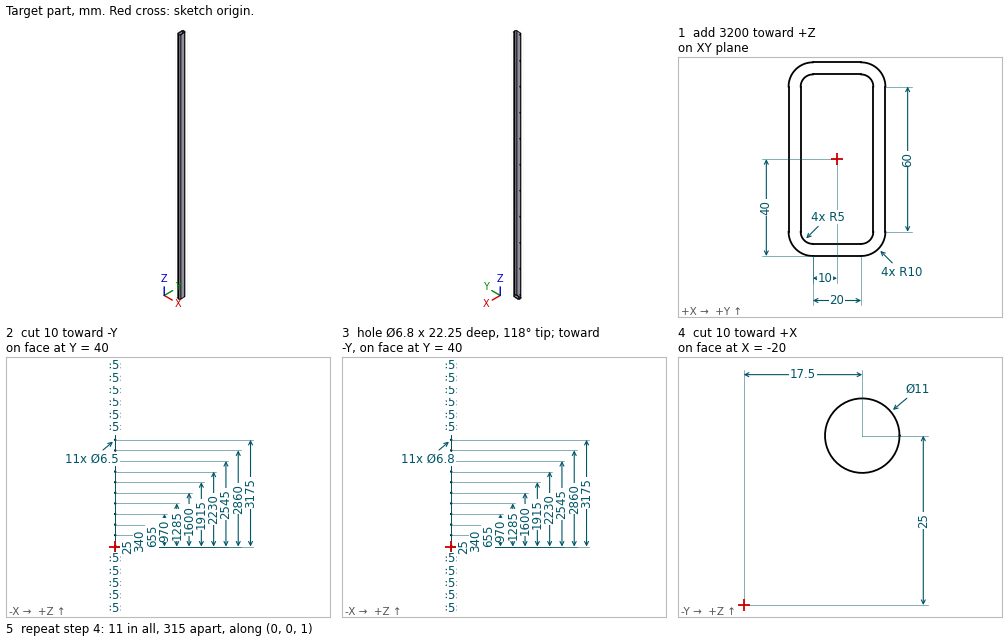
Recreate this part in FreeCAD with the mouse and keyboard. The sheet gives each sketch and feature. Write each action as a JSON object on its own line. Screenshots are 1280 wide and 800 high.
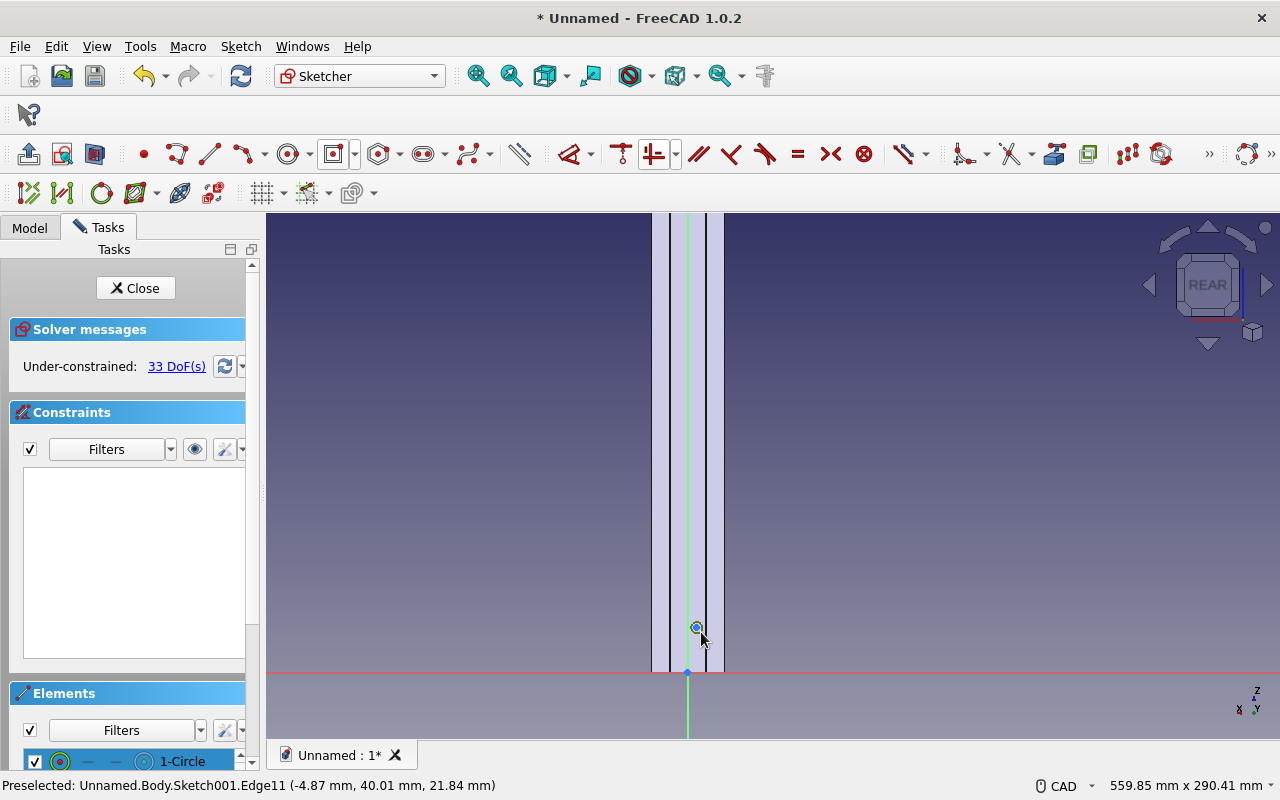
{"action": "key", "text": "e"}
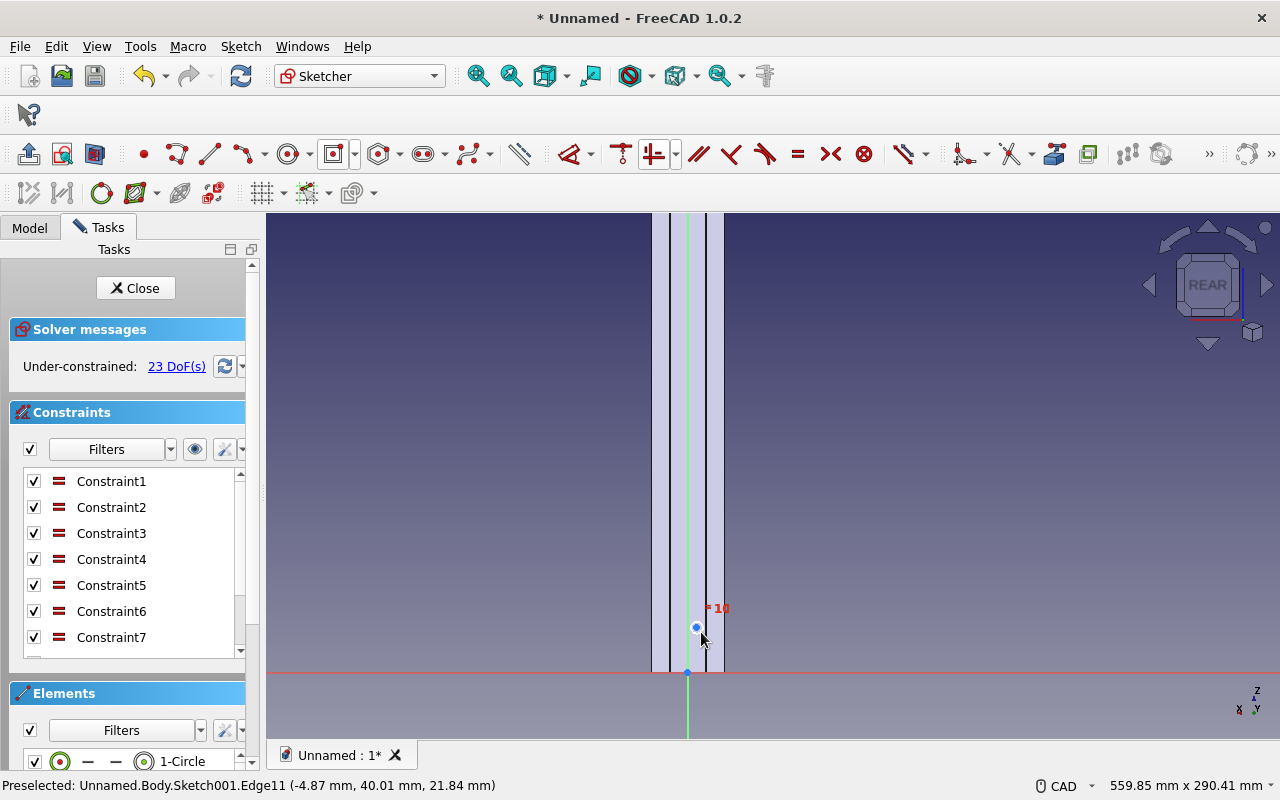
{"action": "left_click", "coordinate": [568, 154]}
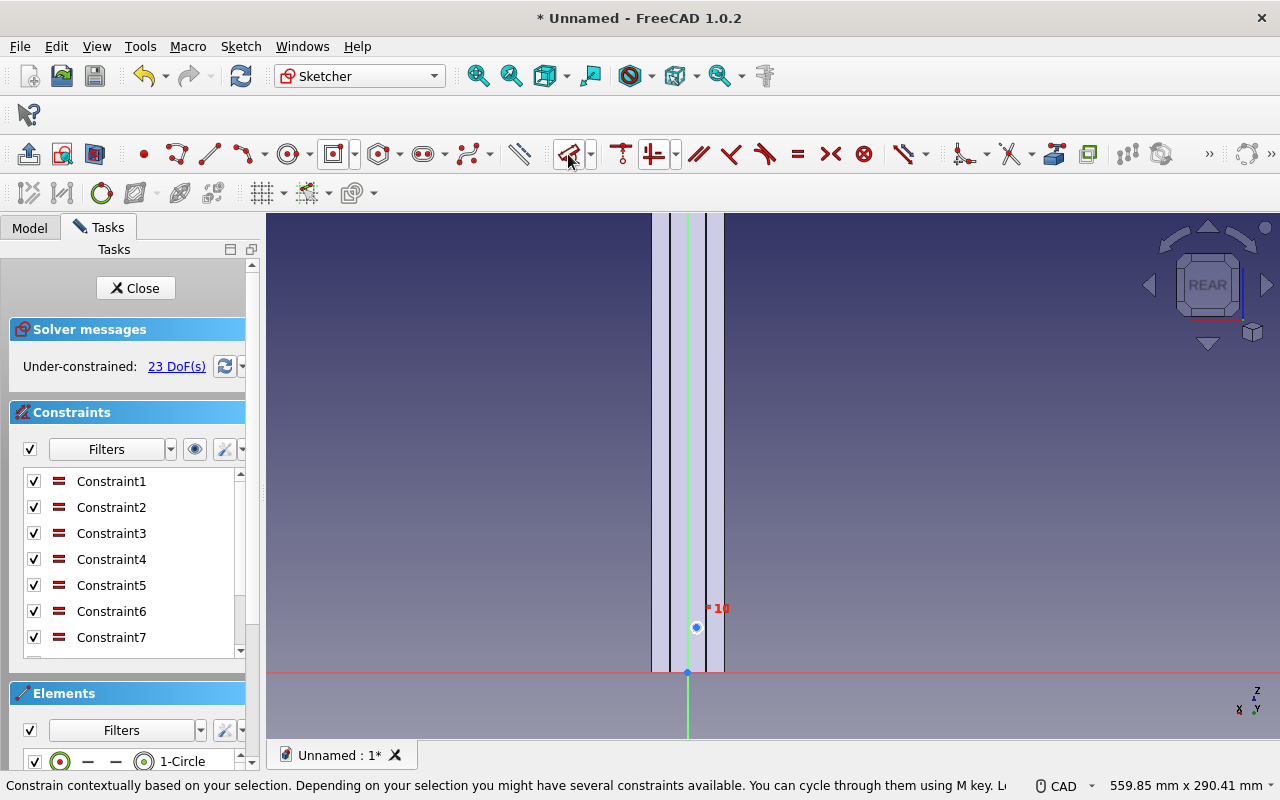
{"action": "scroll", "coordinate": [705, 650], "scroll_direction": "down", "scroll_amount": 14}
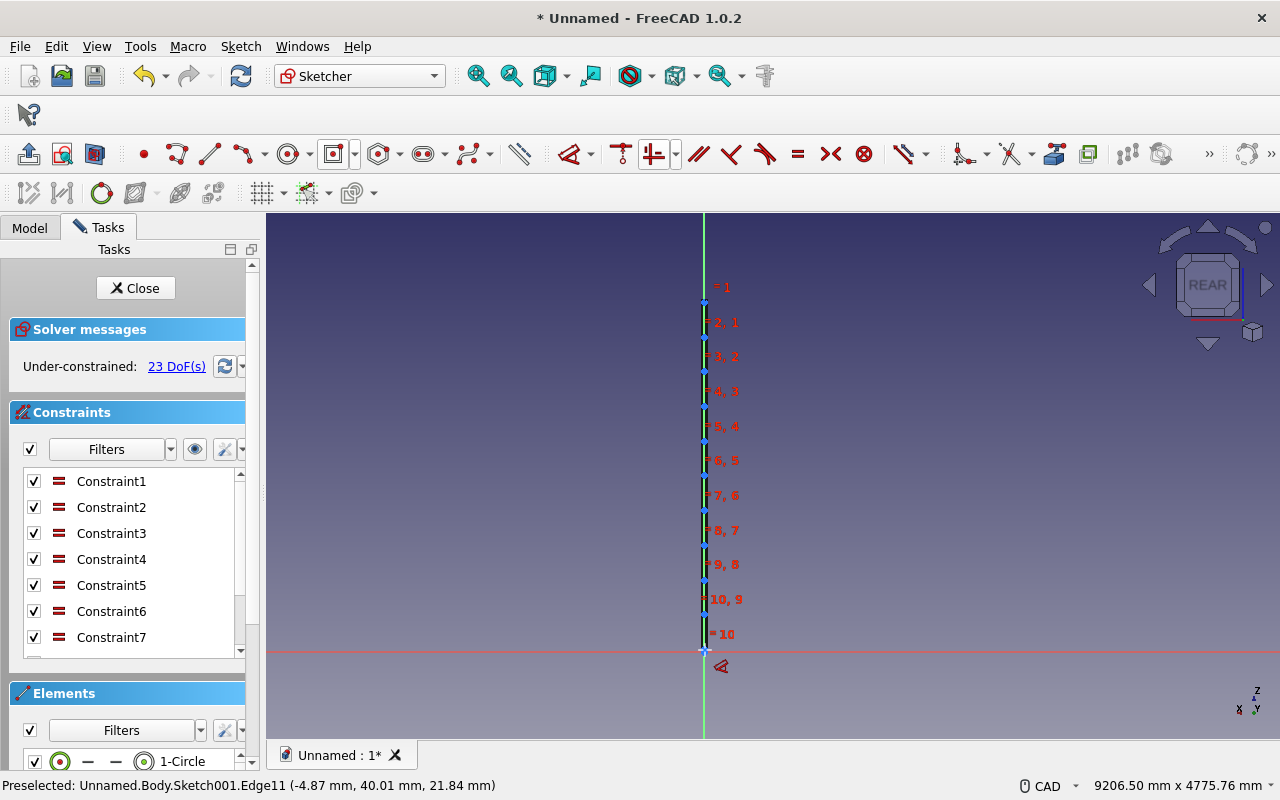
{"action": "scroll", "coordinate": [705, 303], "scroll_direction": "up", "scroll_amount": 21}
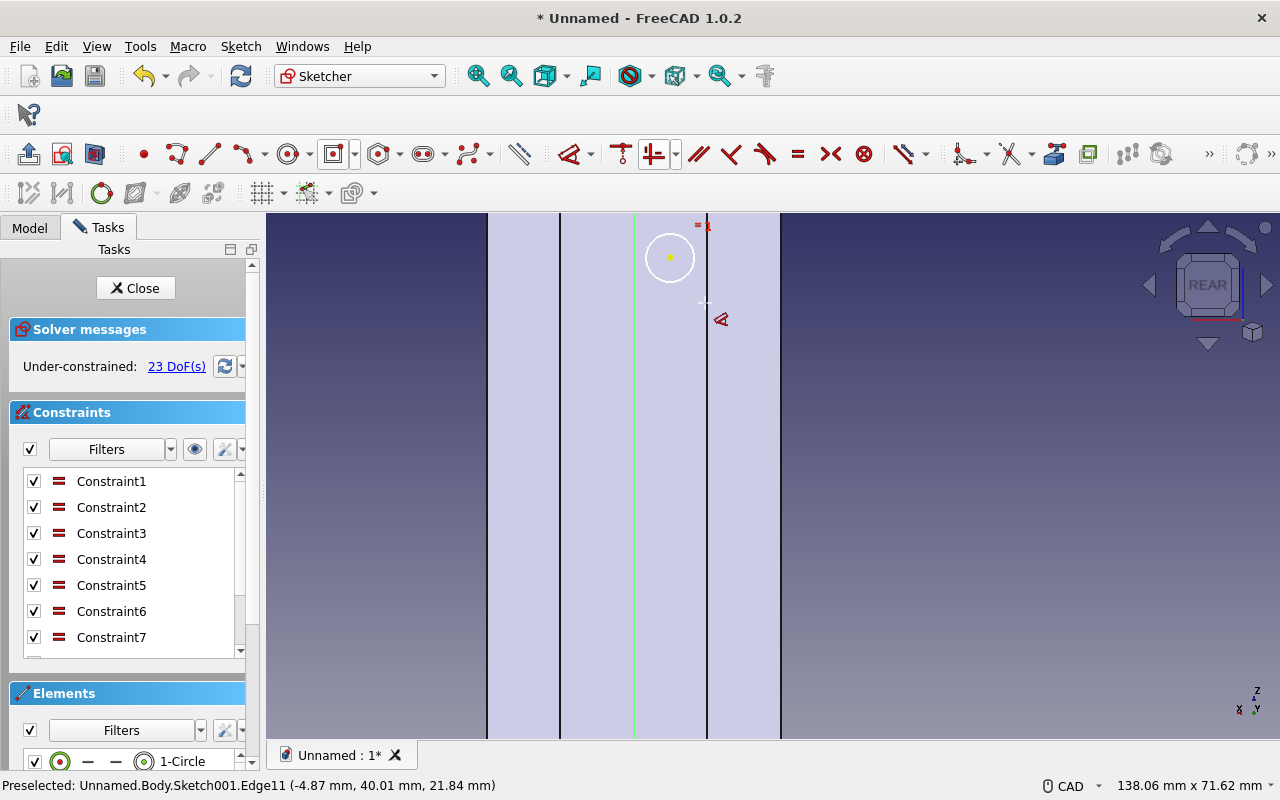
{"action": "left_click", "coordinate": [687, 275]}
{"action": "left_click", "coordinate": [710, 298]}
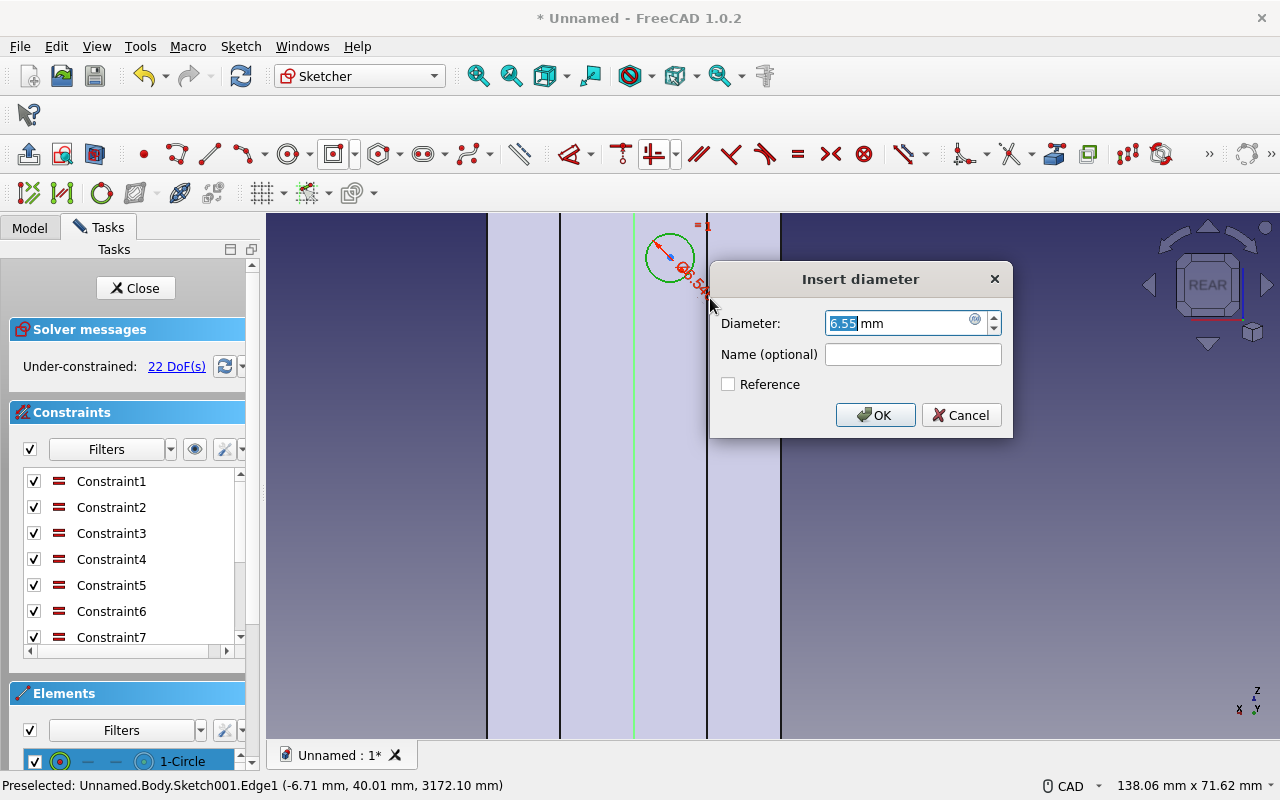
{"action": "type", "text": "6.5"}
{"action": "key", "text": "Return"}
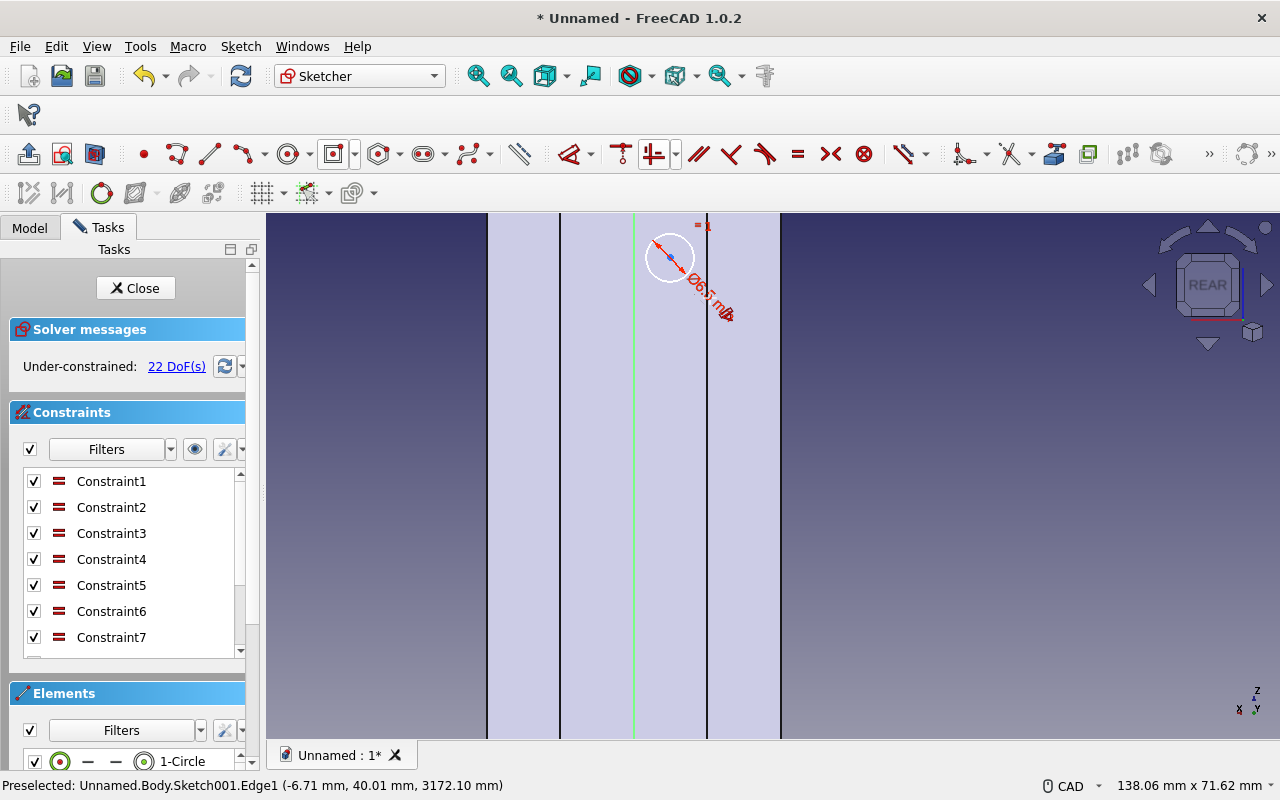
{"action": "left_click", "coordinate": [670, 258]}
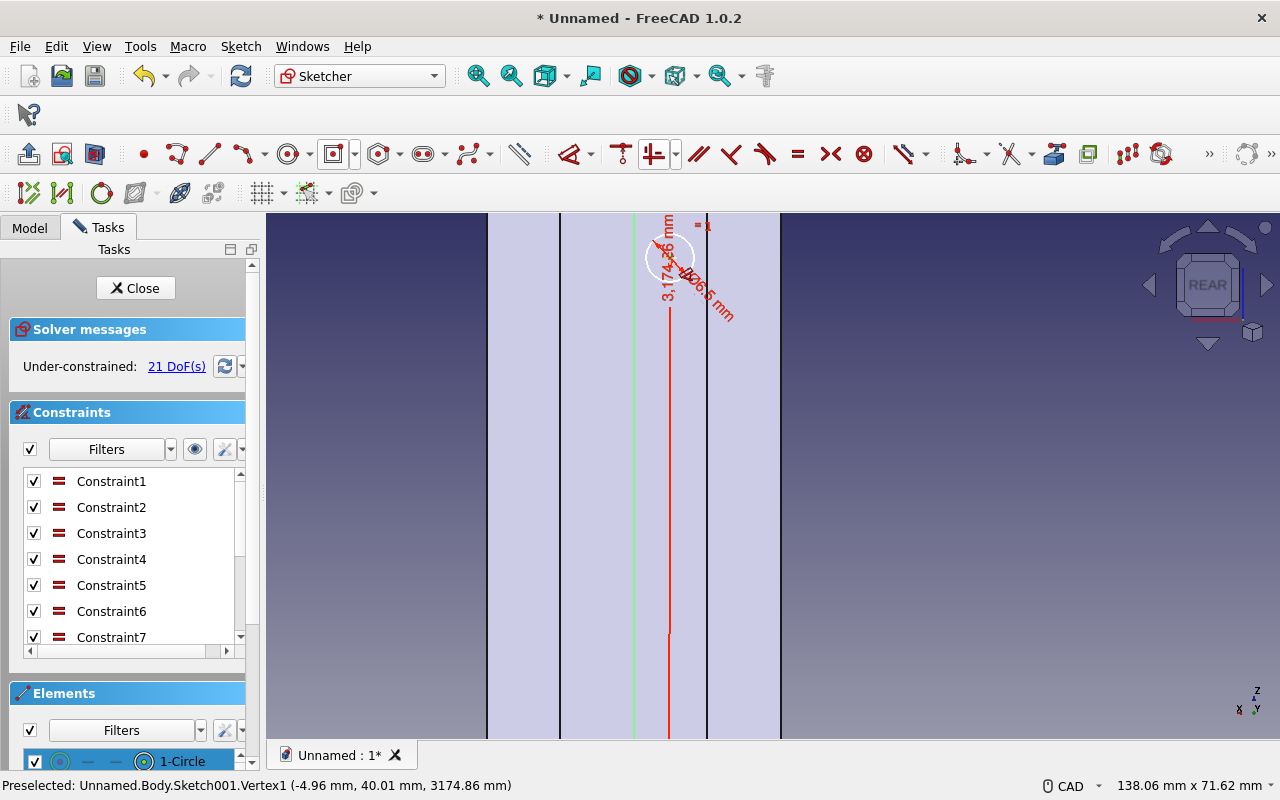
{"action": "key", "text": "Escape"}
{"action": "key", "text": "Escape"}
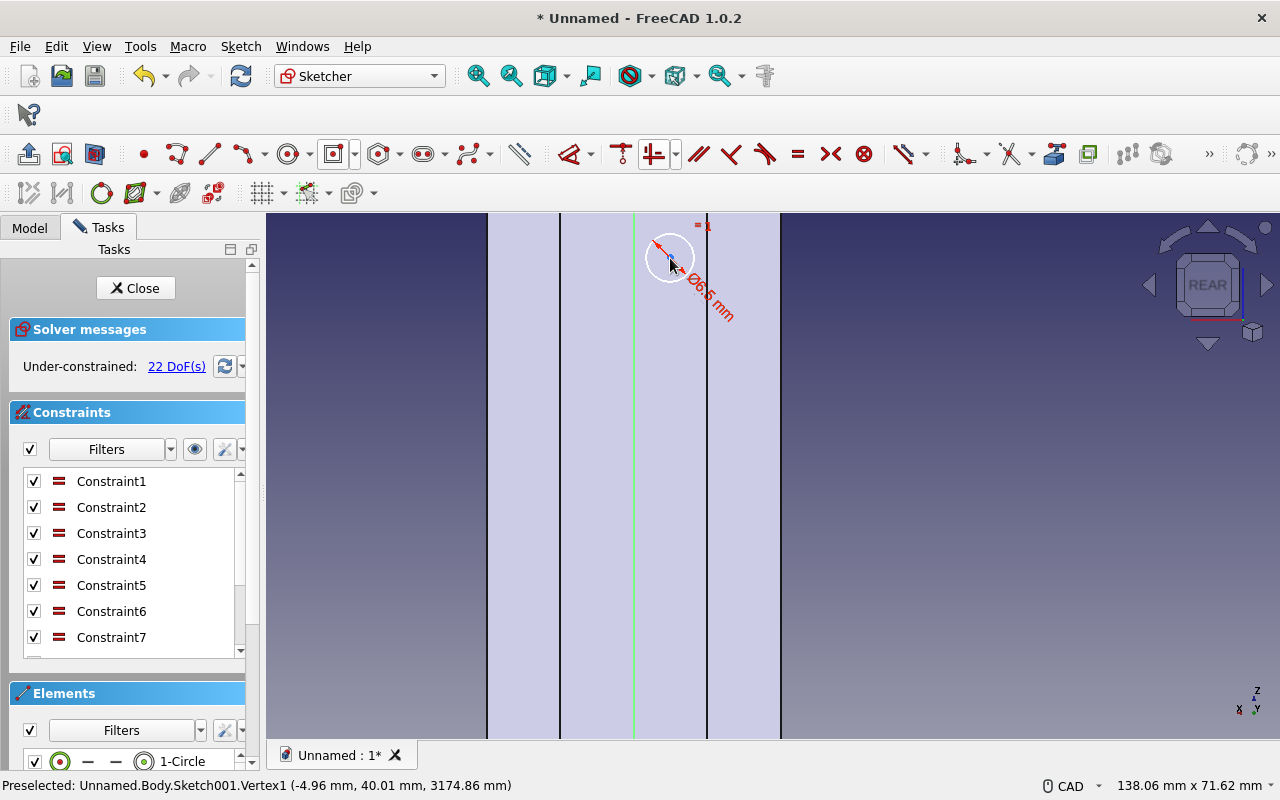
{"action": "left_click", "coordinate": [670, 258]}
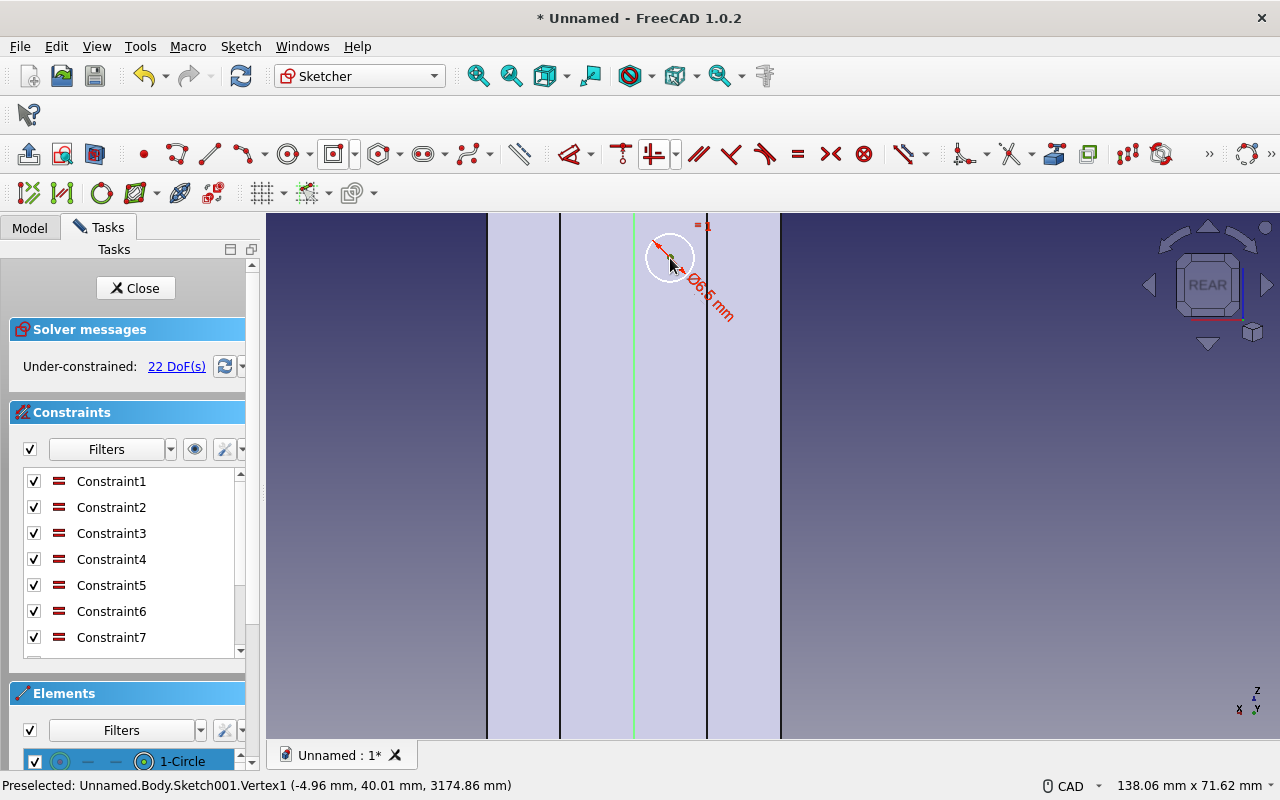
{"action": "key", "text": "l"}